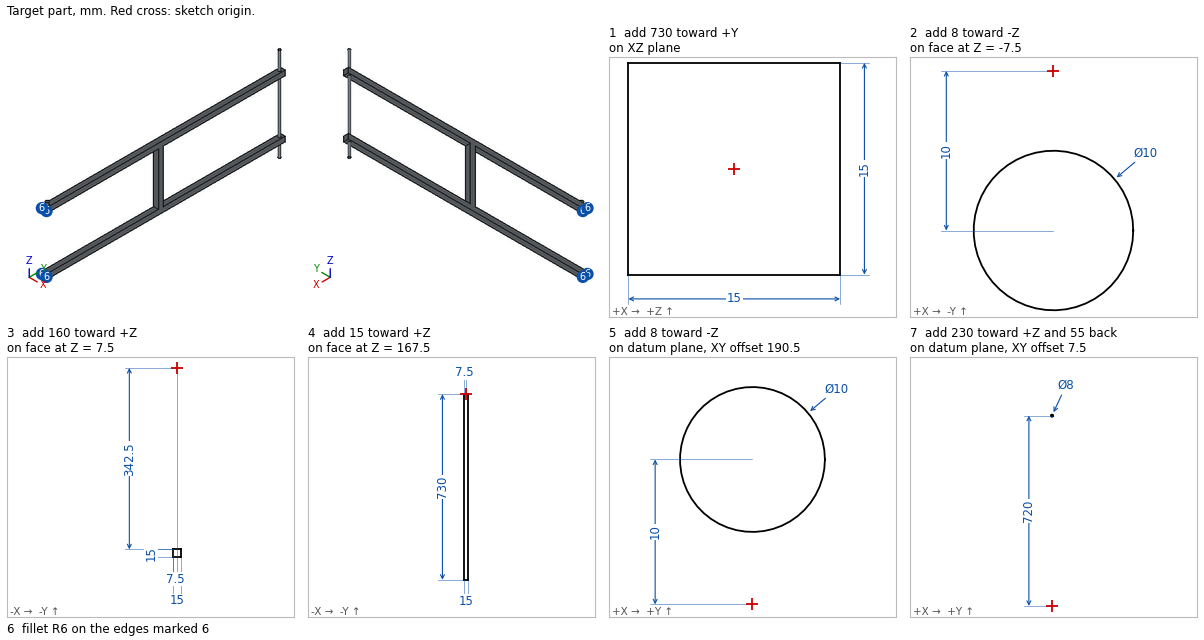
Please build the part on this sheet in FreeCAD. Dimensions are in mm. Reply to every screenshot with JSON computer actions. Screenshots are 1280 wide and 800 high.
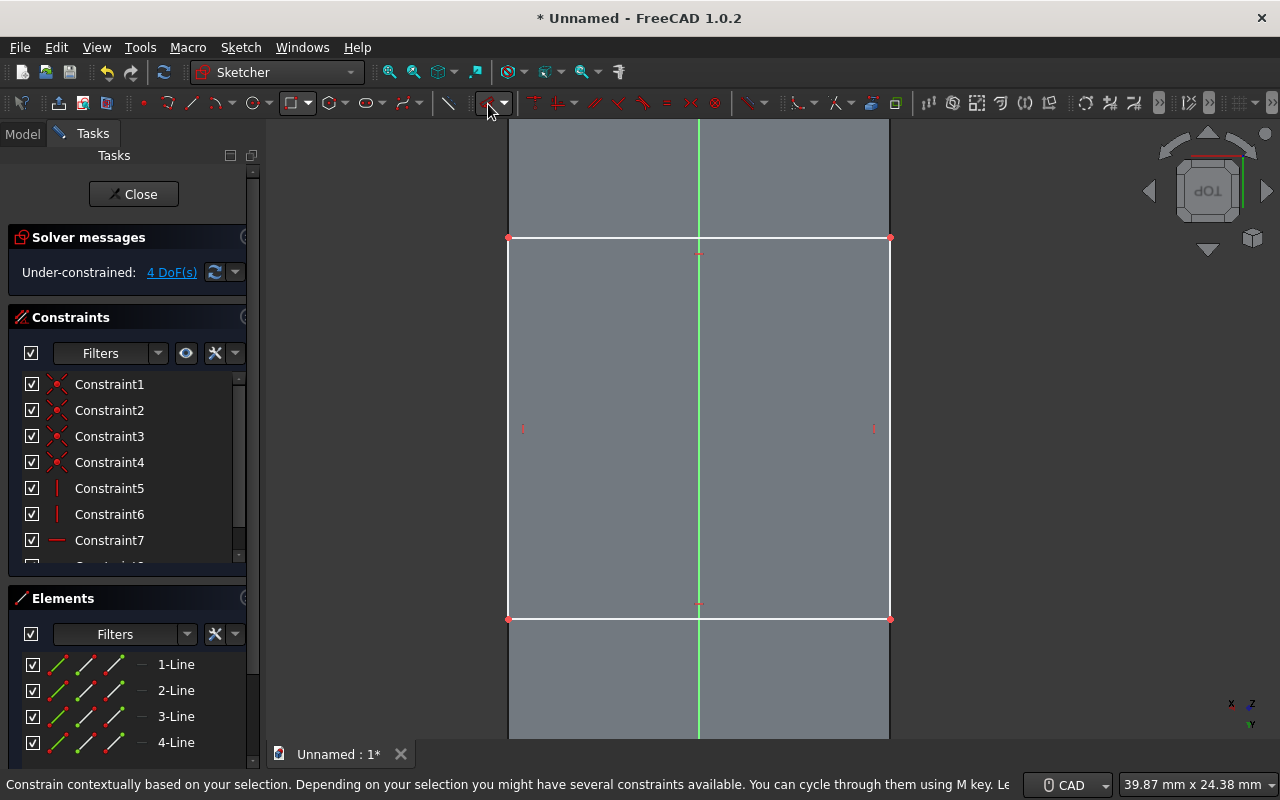
{"action": "left_click", "coordinate": [508, 352]}
{"action": "left_click", "coordinate": [474, 429]}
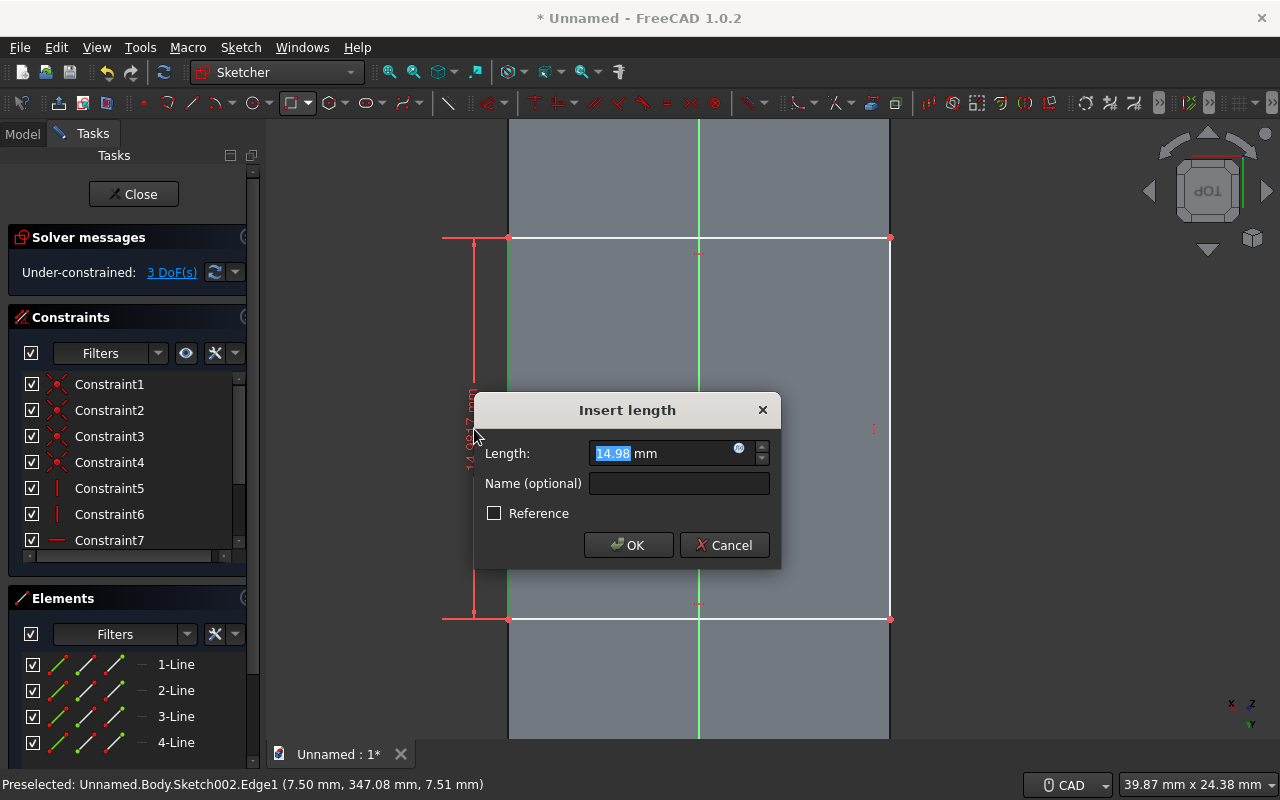
{"action": "type", "text": "15"}
{"action": "key", "text": "Return"}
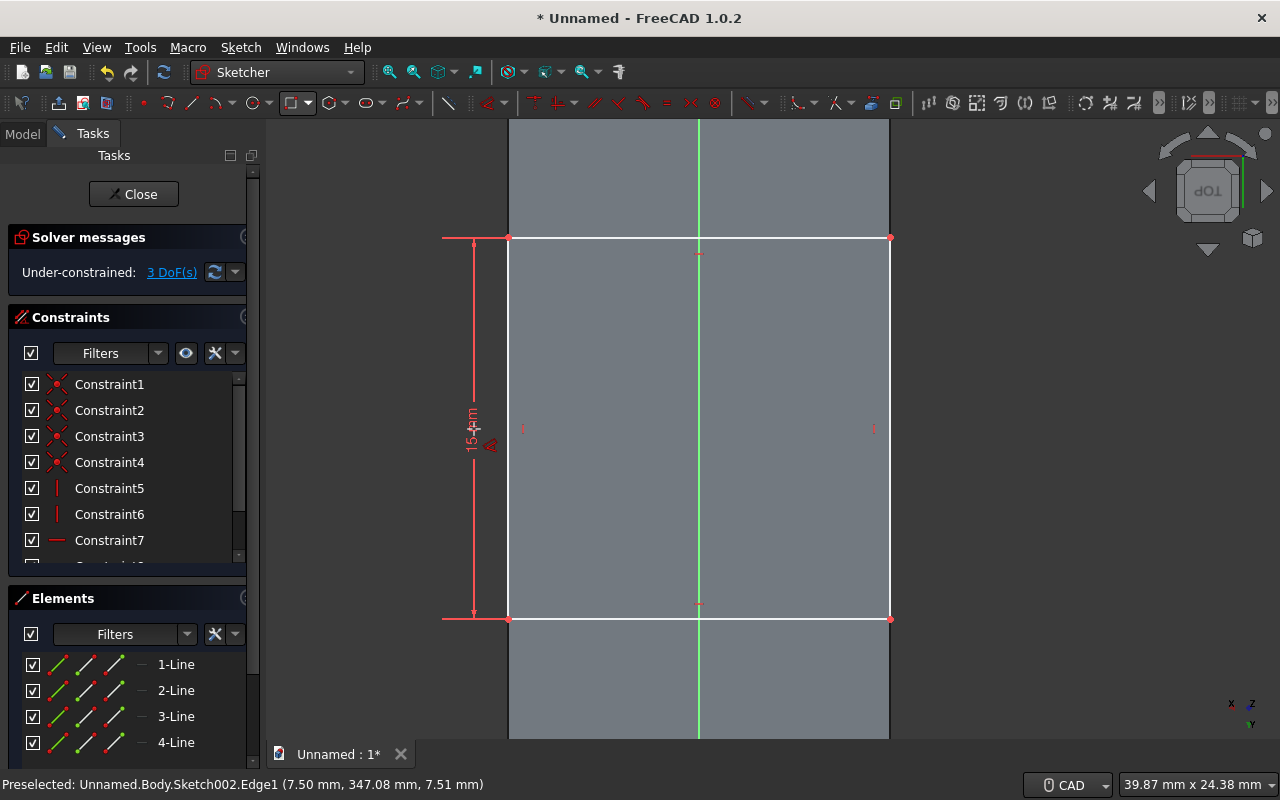
{"action": "left_click", "coordinate": [623, 619]}
{"action": "left_click", "coordinate": [611, 653]}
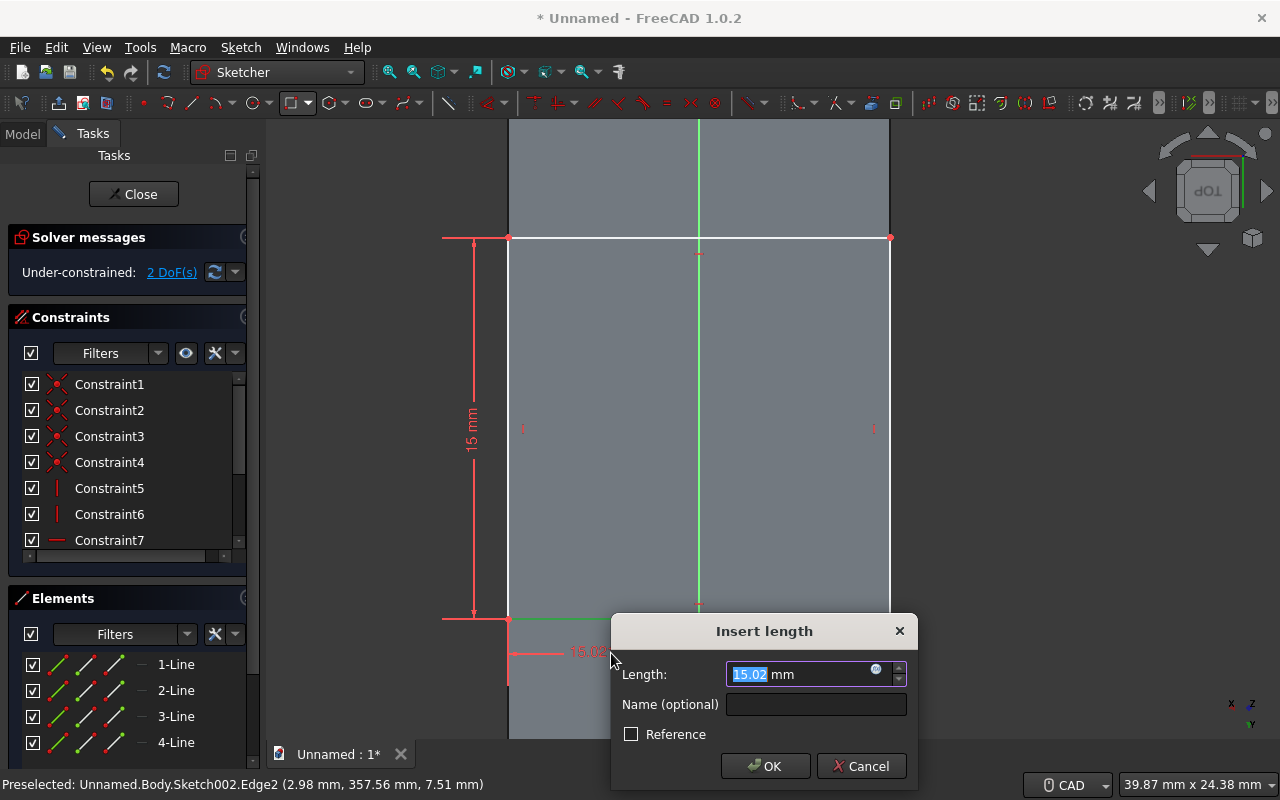
{"action": "type", "text": "15"}
{"action": "key", "text": "Return"}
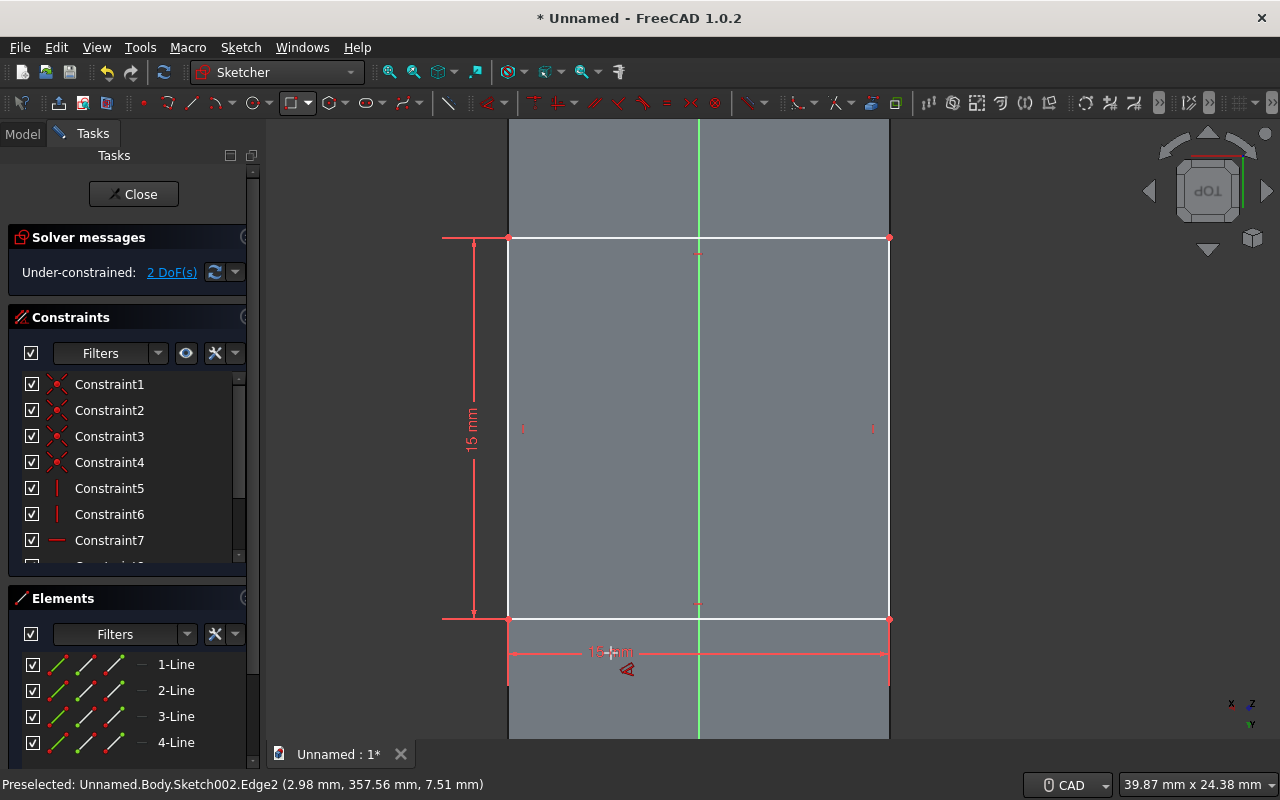
{"action": "left_click", "coordinate": [508, 238]}
{"action": "left_click", "coordinate": [603, 272]}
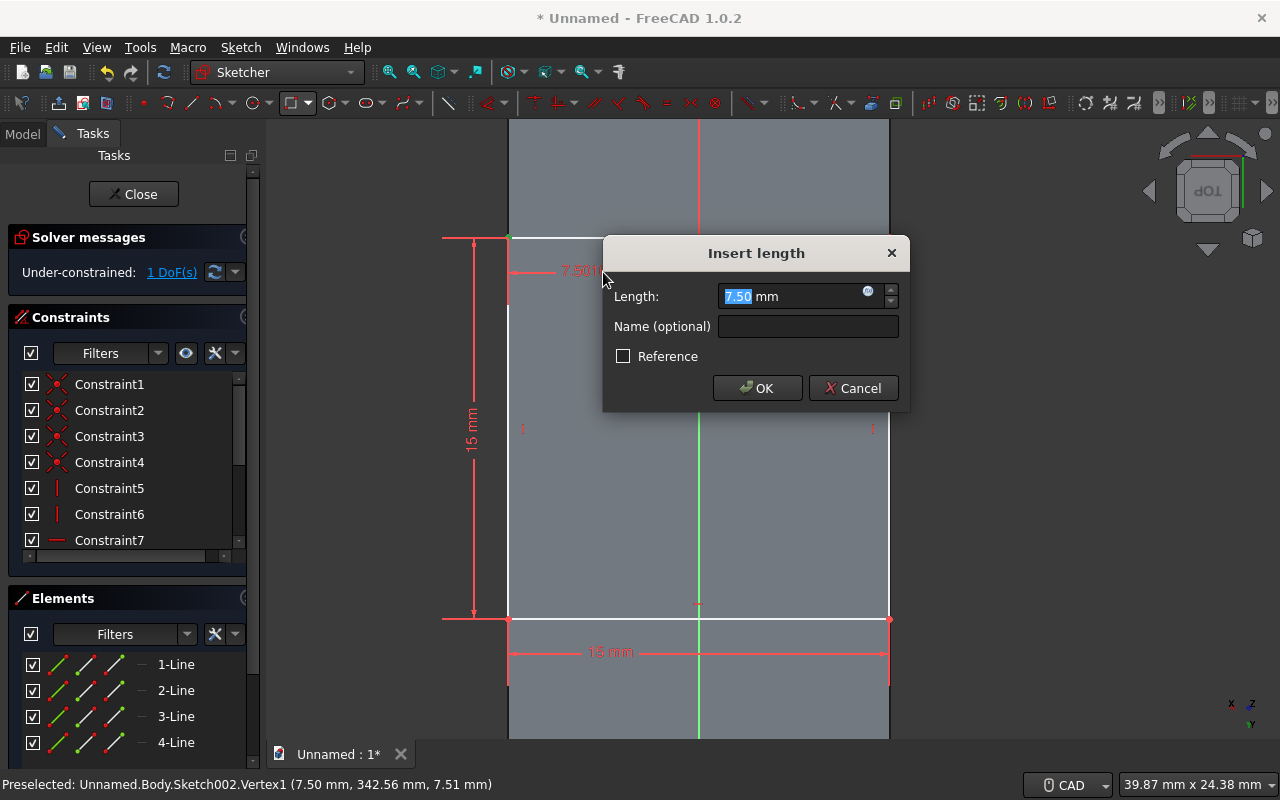
{"action": "type", "text": "7.5"}
{"action": "key", "text": "Return"}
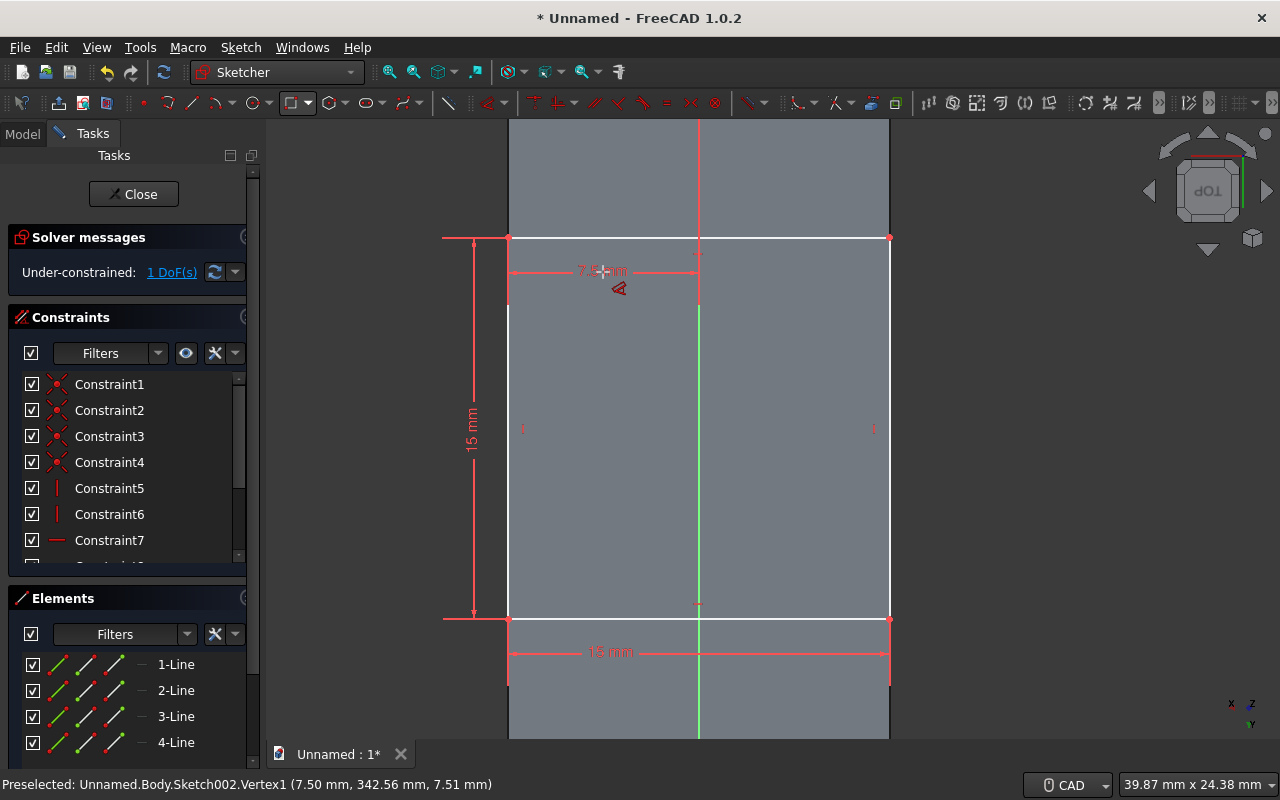
{"action": "left_click", "coordinate": [508, 238]}
{"action": "left_click", "coordinate": [474, 193]}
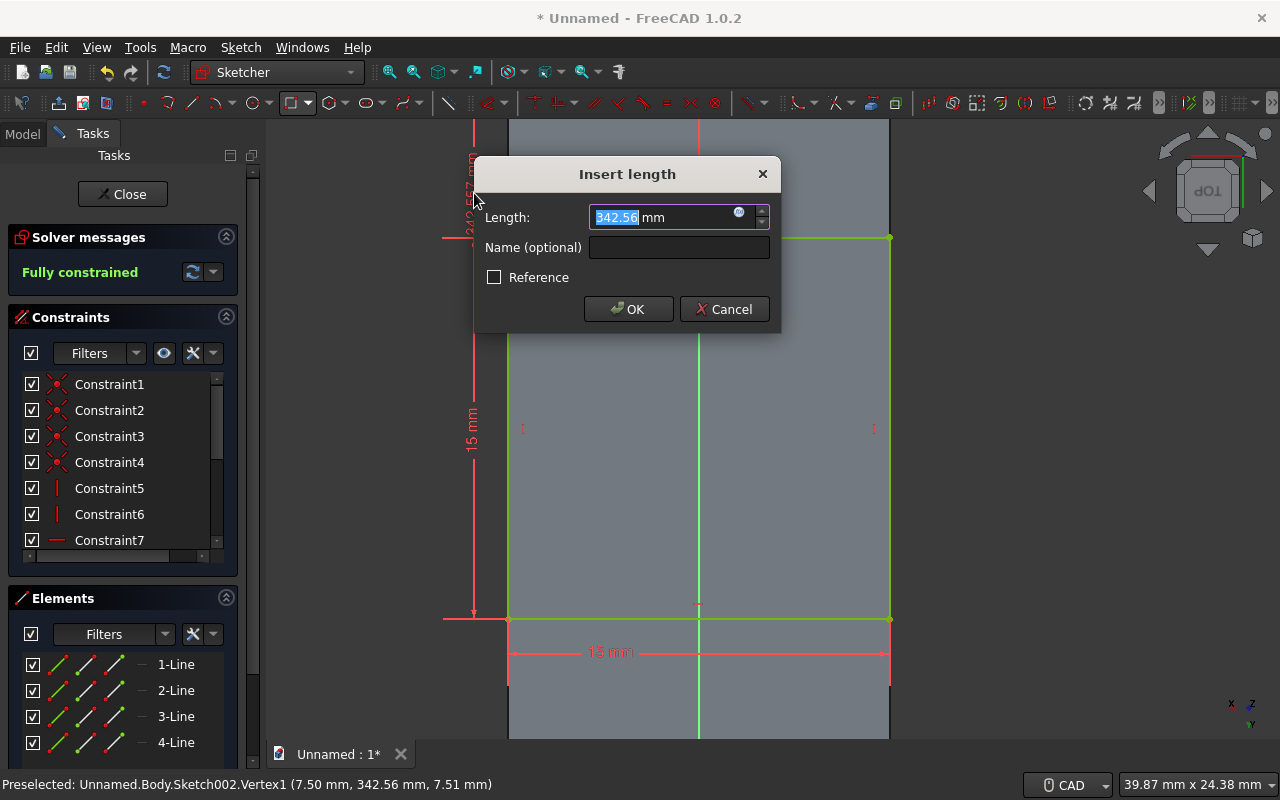
{"action": "type", "text": "342.5"}
{"action": "key", "text": "Return"}
{"action": "key", "text": "Escape"}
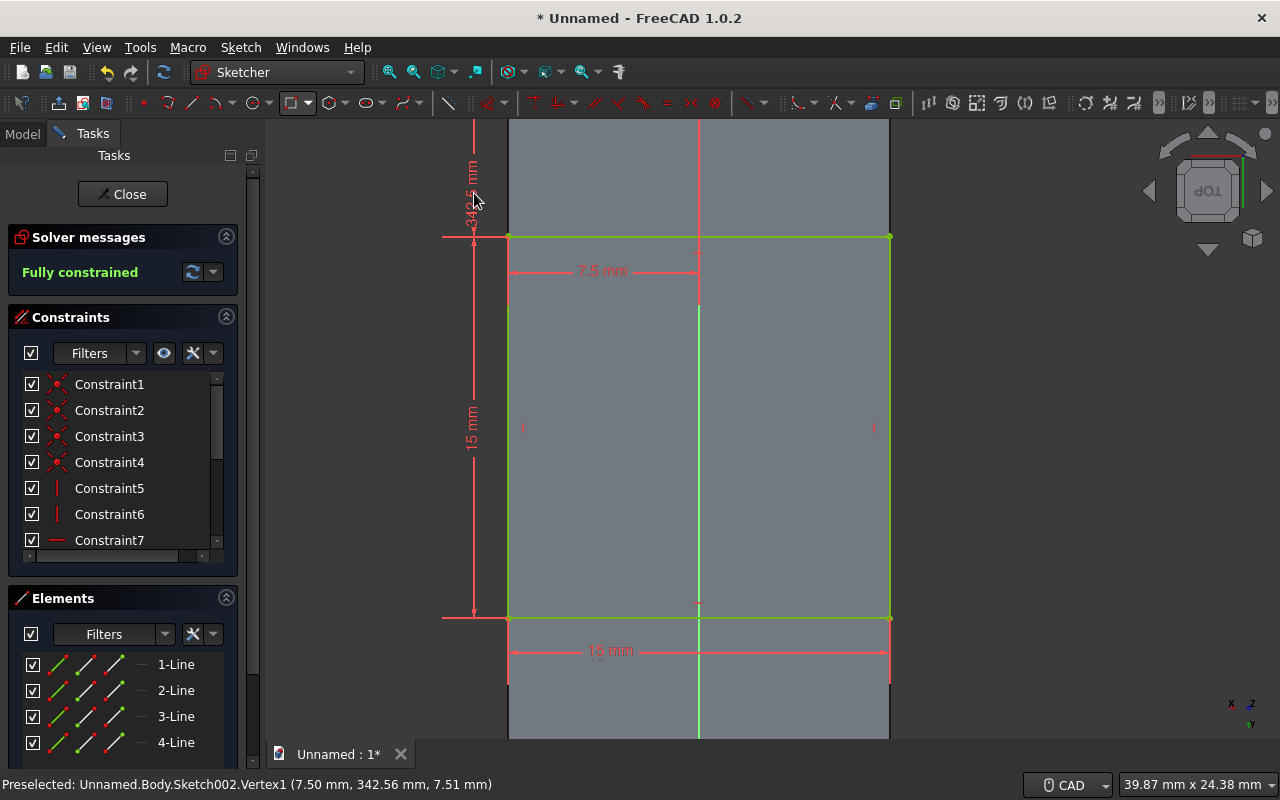
{"action": "left_click", "coordinate": [123, 194]}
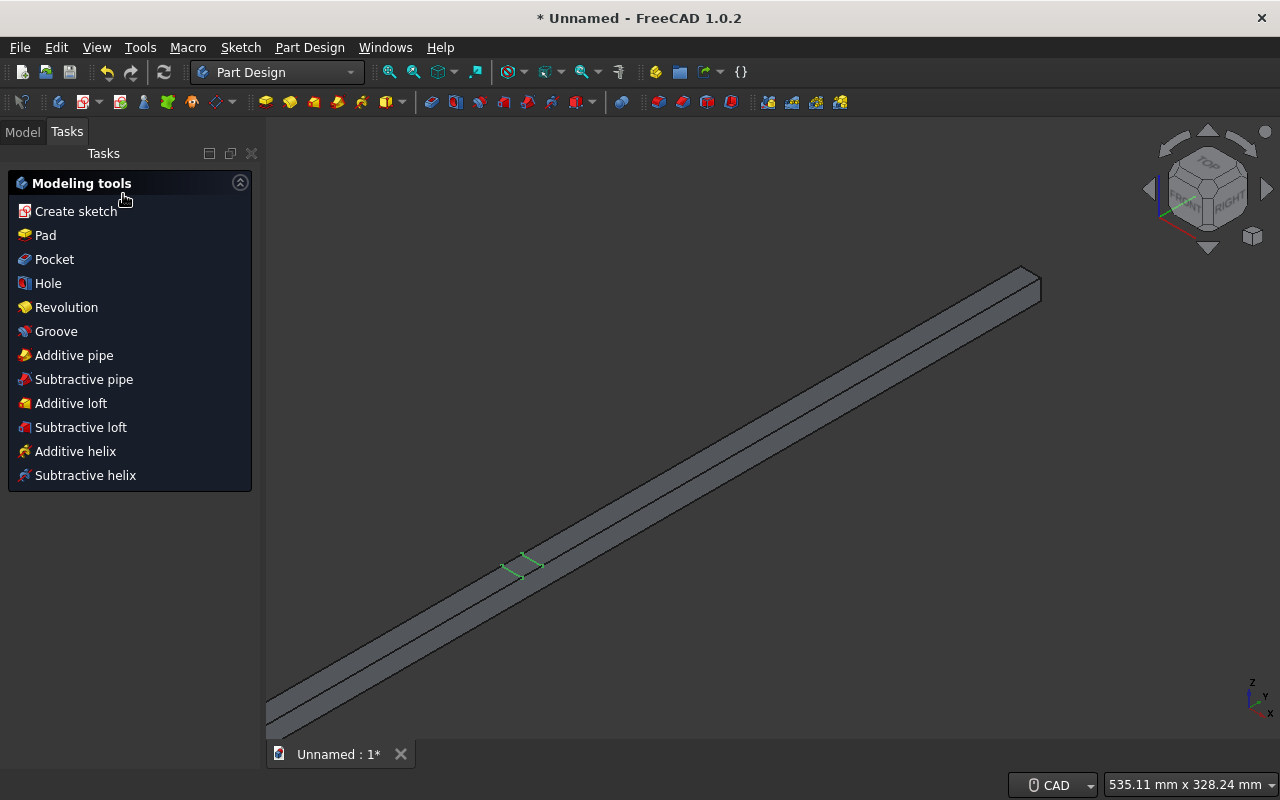
{"action": "left_click", "coordinate": [266, 102]}